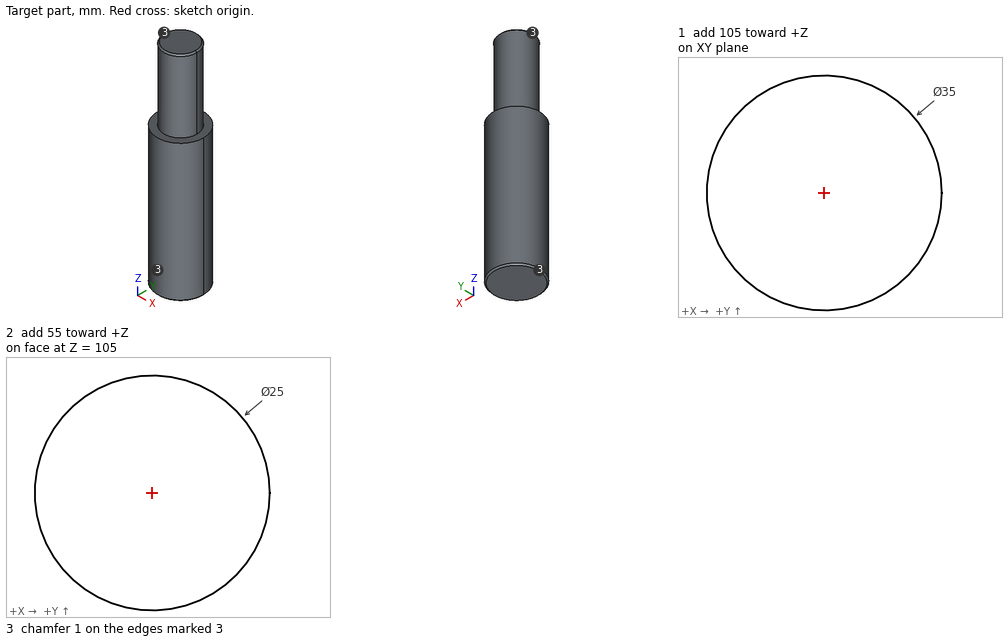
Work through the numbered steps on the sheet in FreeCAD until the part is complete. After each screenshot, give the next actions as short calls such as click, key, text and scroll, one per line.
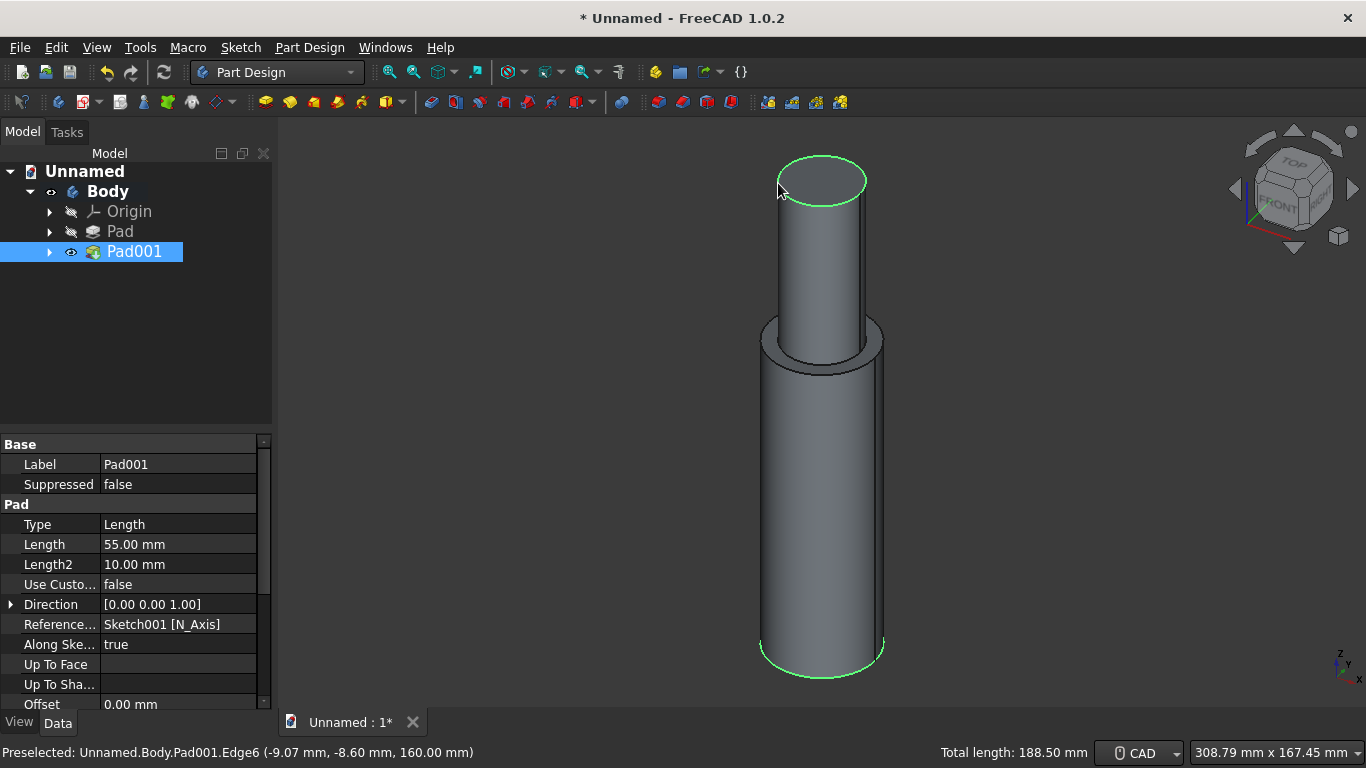
click(684, 102)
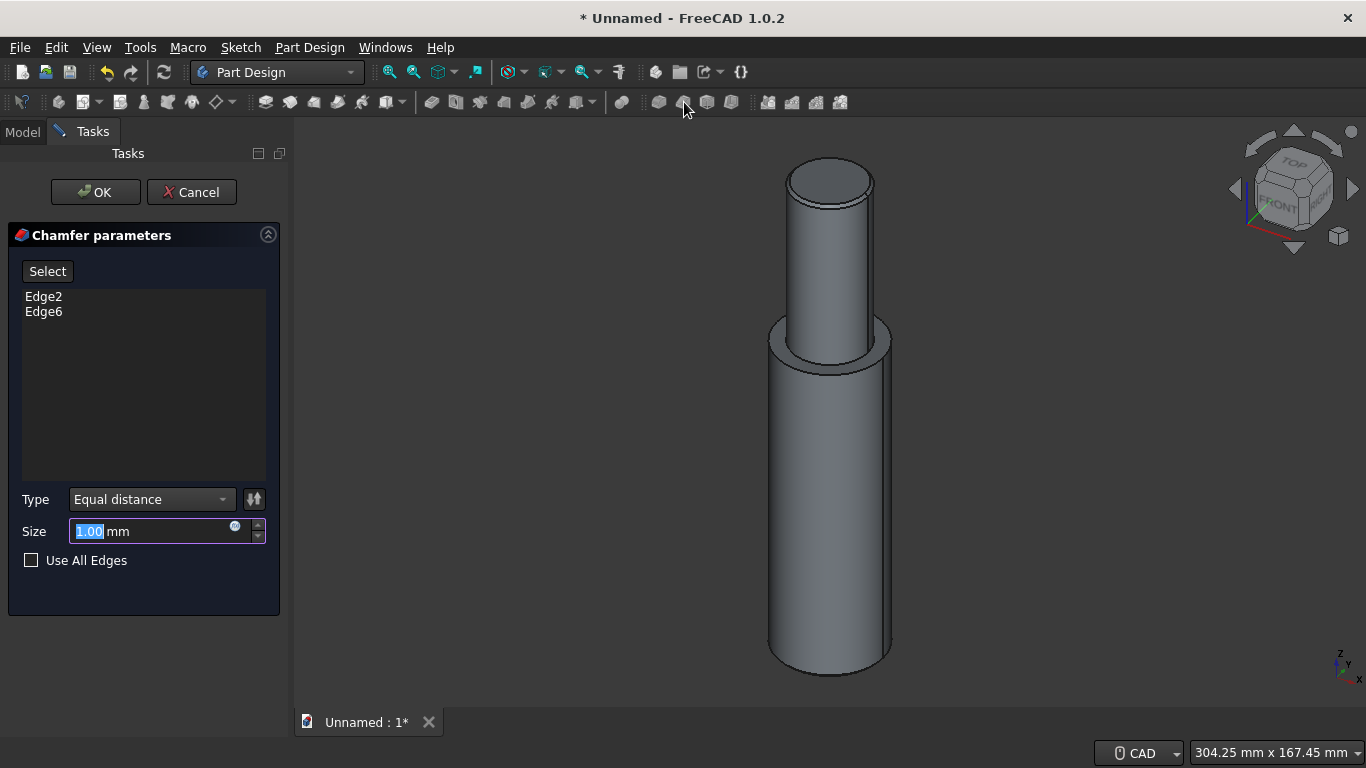
text(1)
key(Tab)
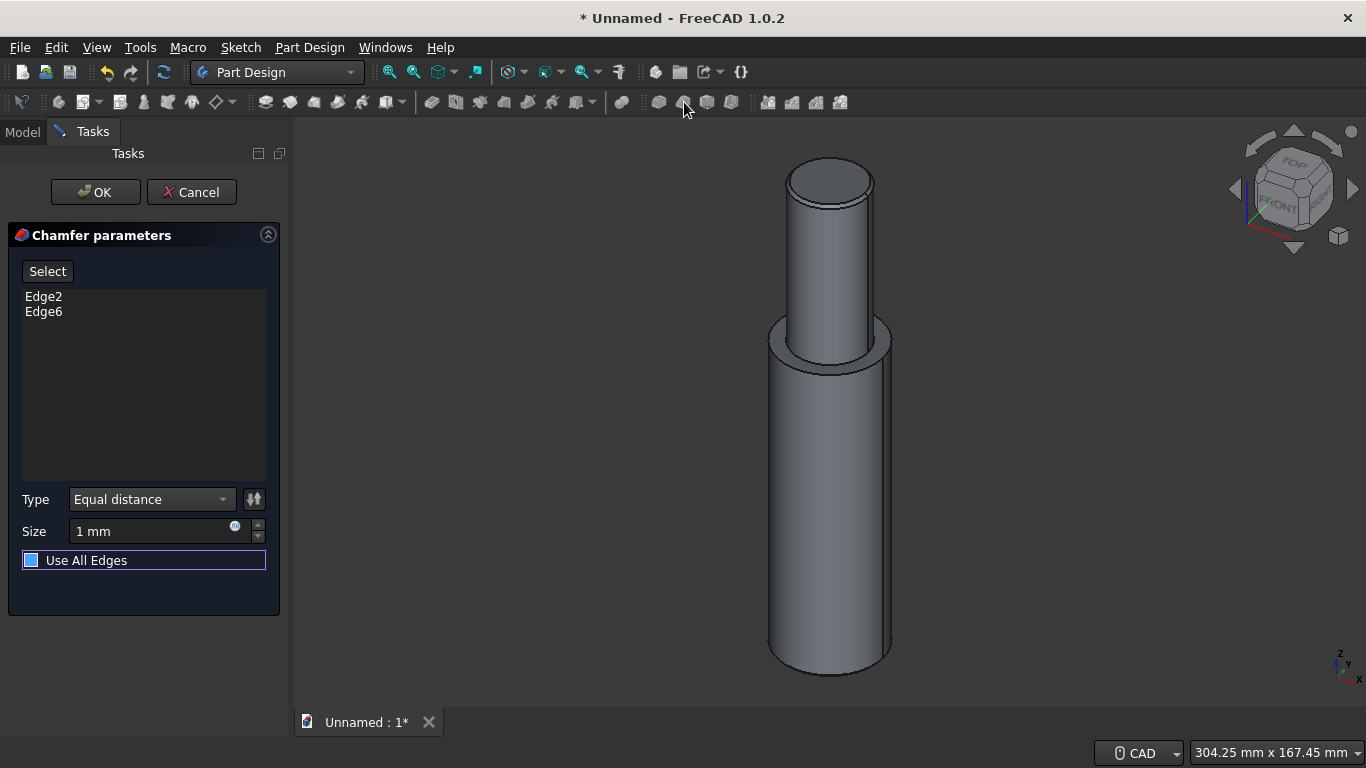
click(96, 192)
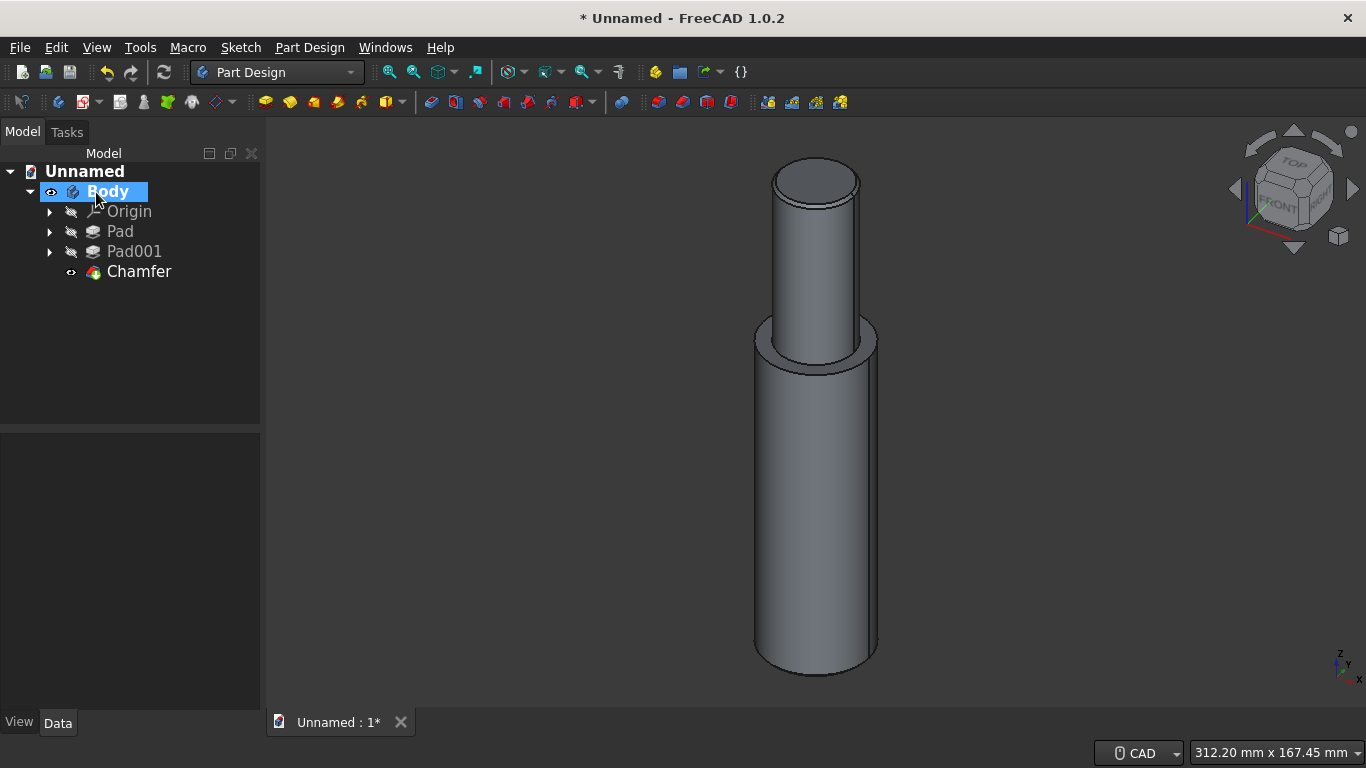
key(0)